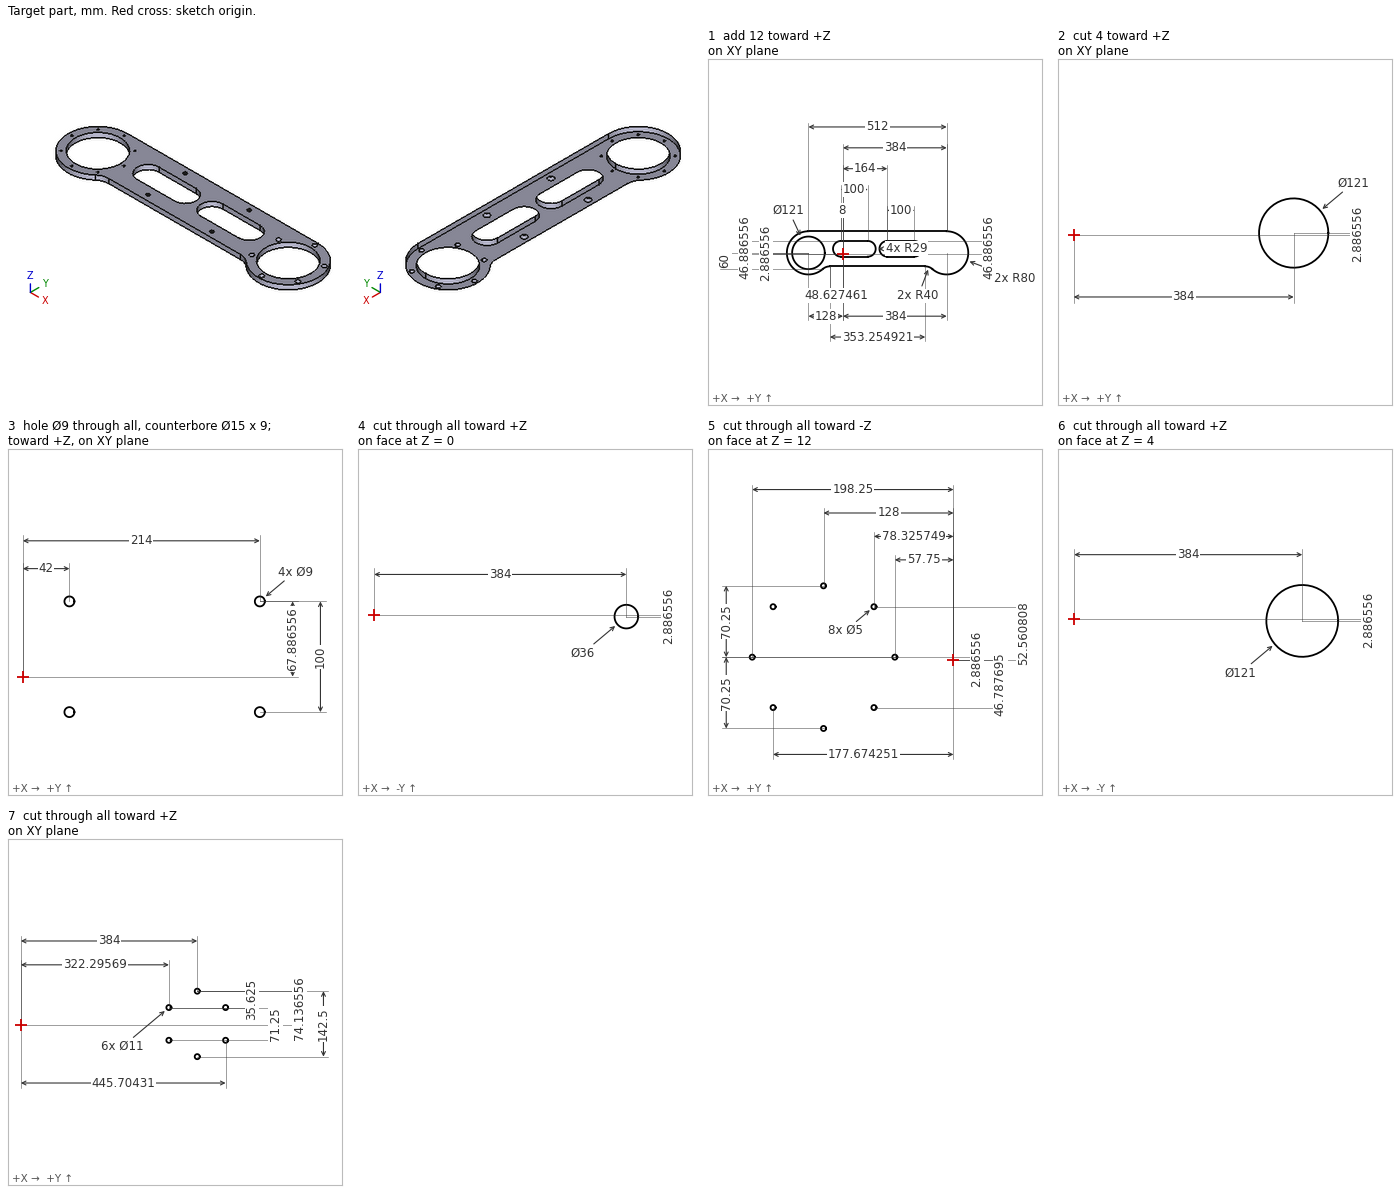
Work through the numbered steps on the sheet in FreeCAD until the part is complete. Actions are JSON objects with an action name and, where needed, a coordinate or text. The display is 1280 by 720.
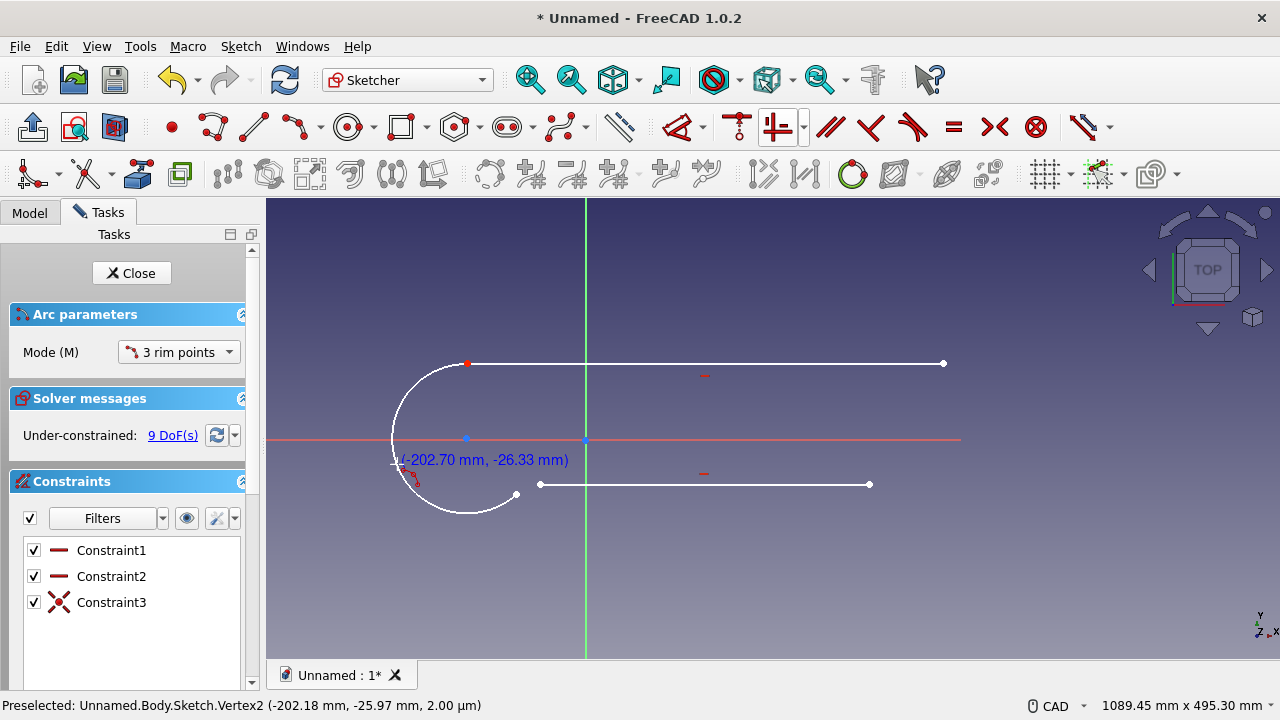
{"action": "left_click", "coordinate": [516, 495]}
{"action": "left_click", "coordinate": [540, 485]}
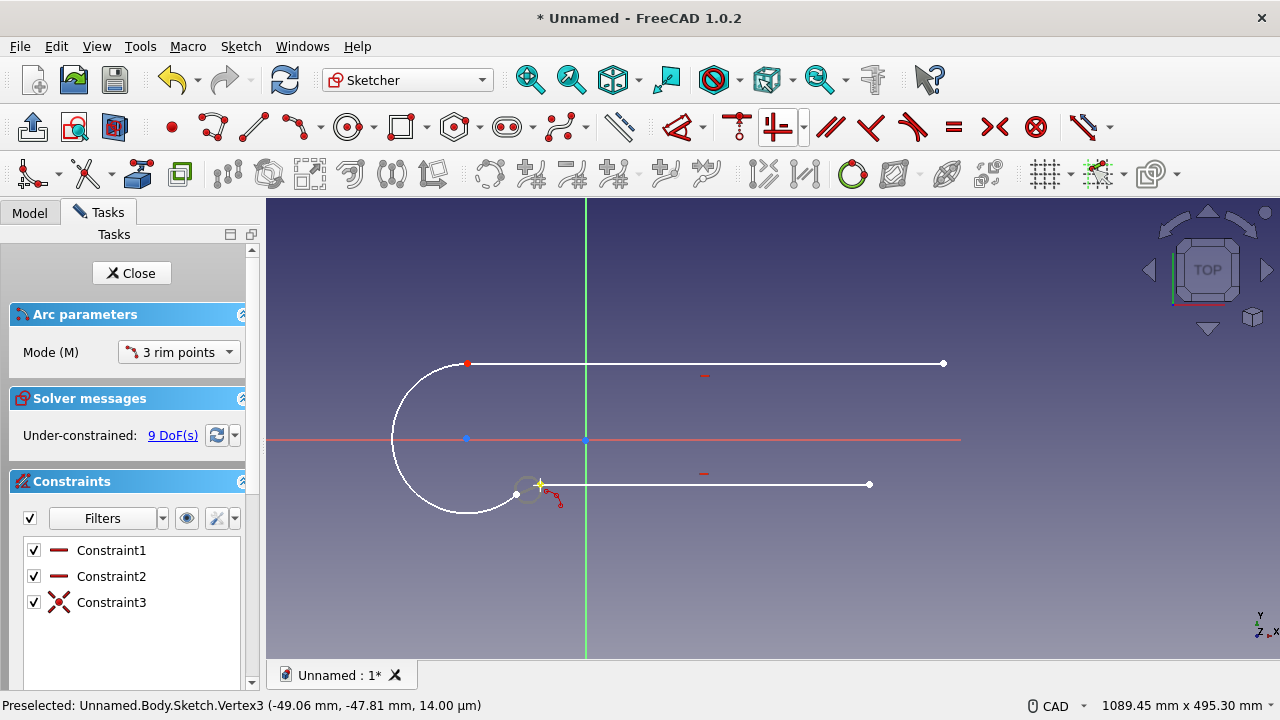
{"action": "scroll", "coordinate": [527, 487], "scroll_direction": "up", "scroll_amount": 10}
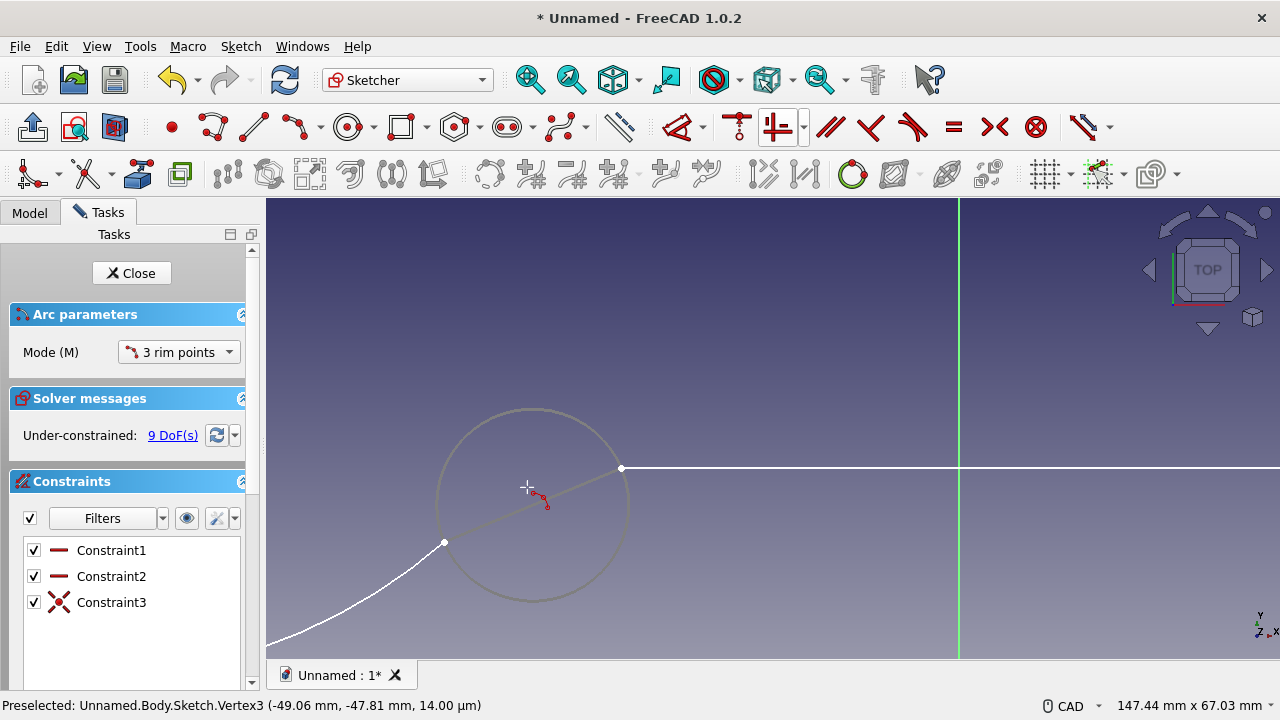
{"action": "left_click", "coordinate": [527, 481]}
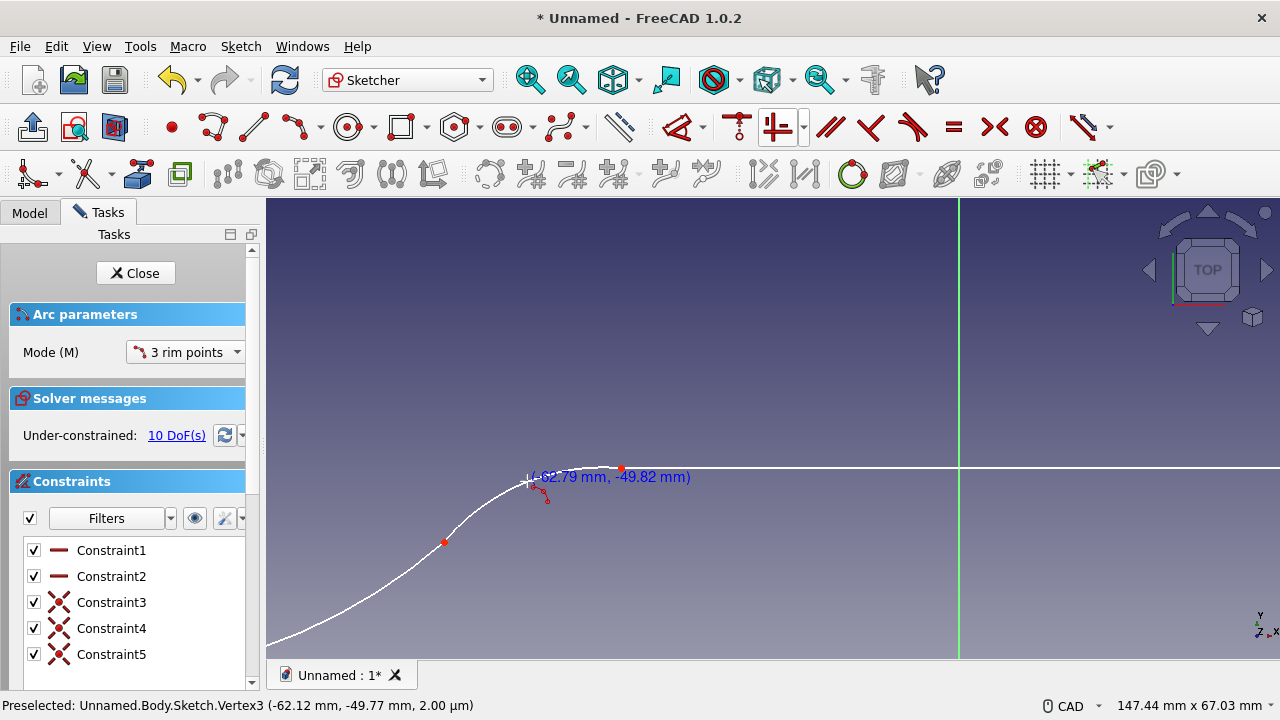
{"action": "scroll", "coordinate": [527, 487], "scroll_direction": "down", "scroll_amount": 10}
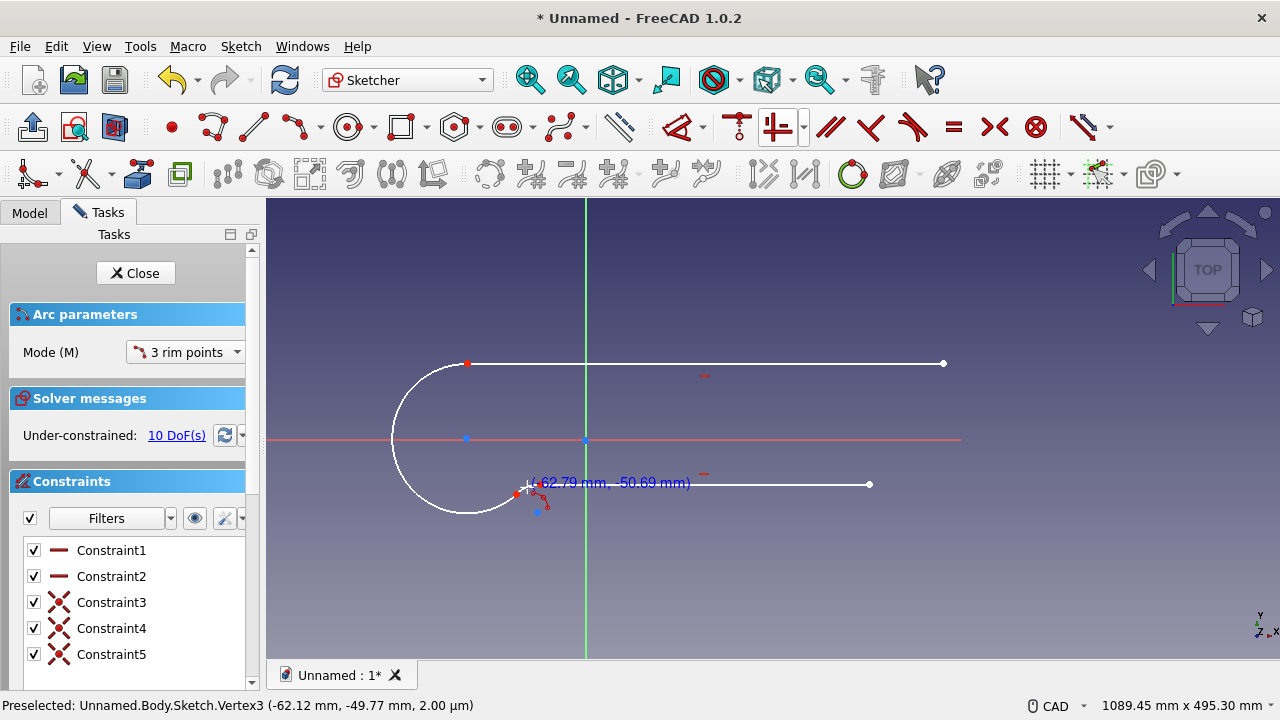
{"action": "left_click", "coordinate": [869, 485]}
{"action": "left_click", "coordinate": [894, 494]}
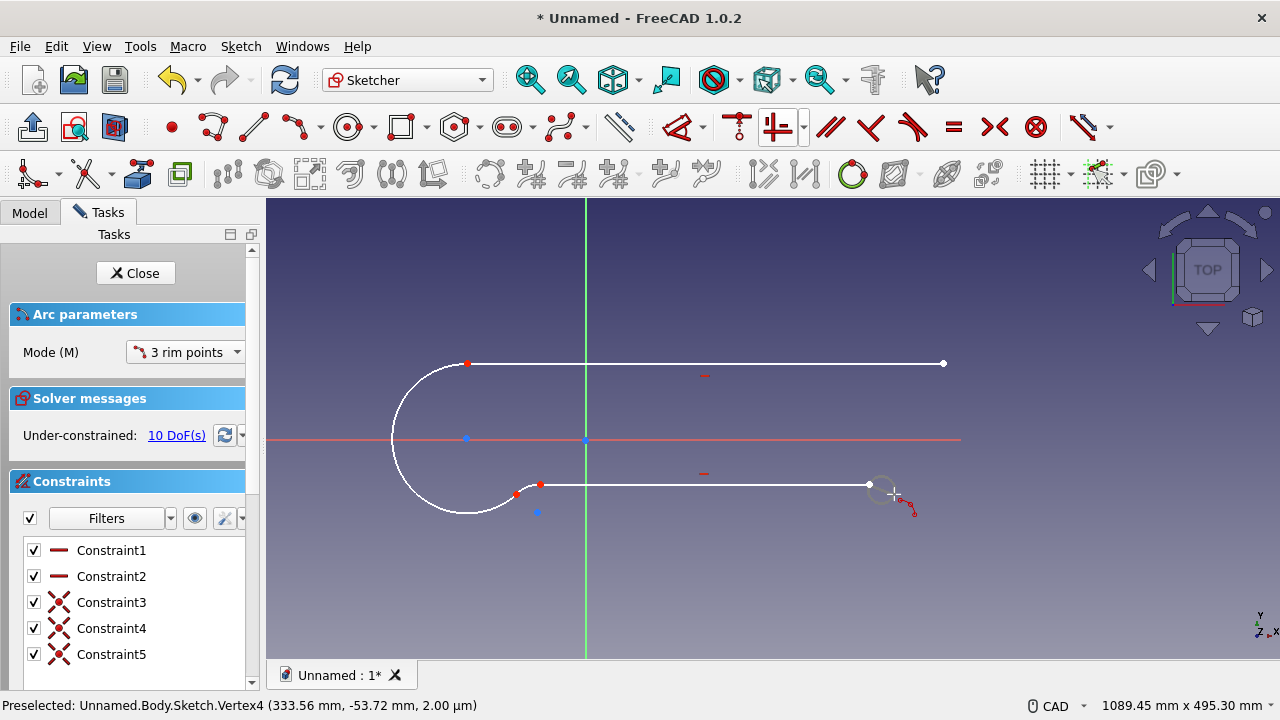
{"action": "scroll", "coordinate": [882, 487], "scroll_direction": "up", "scroll_amount": 10}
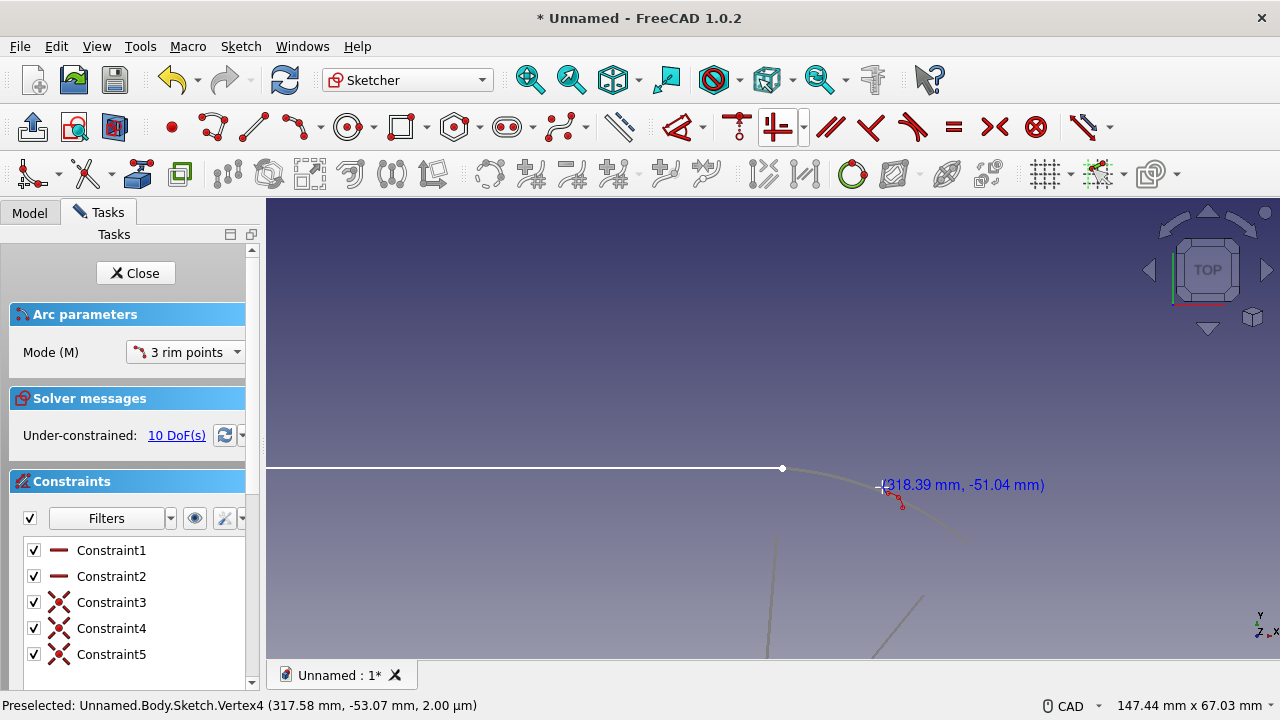
{"action": "left_click", "coordinate": [881, 481]}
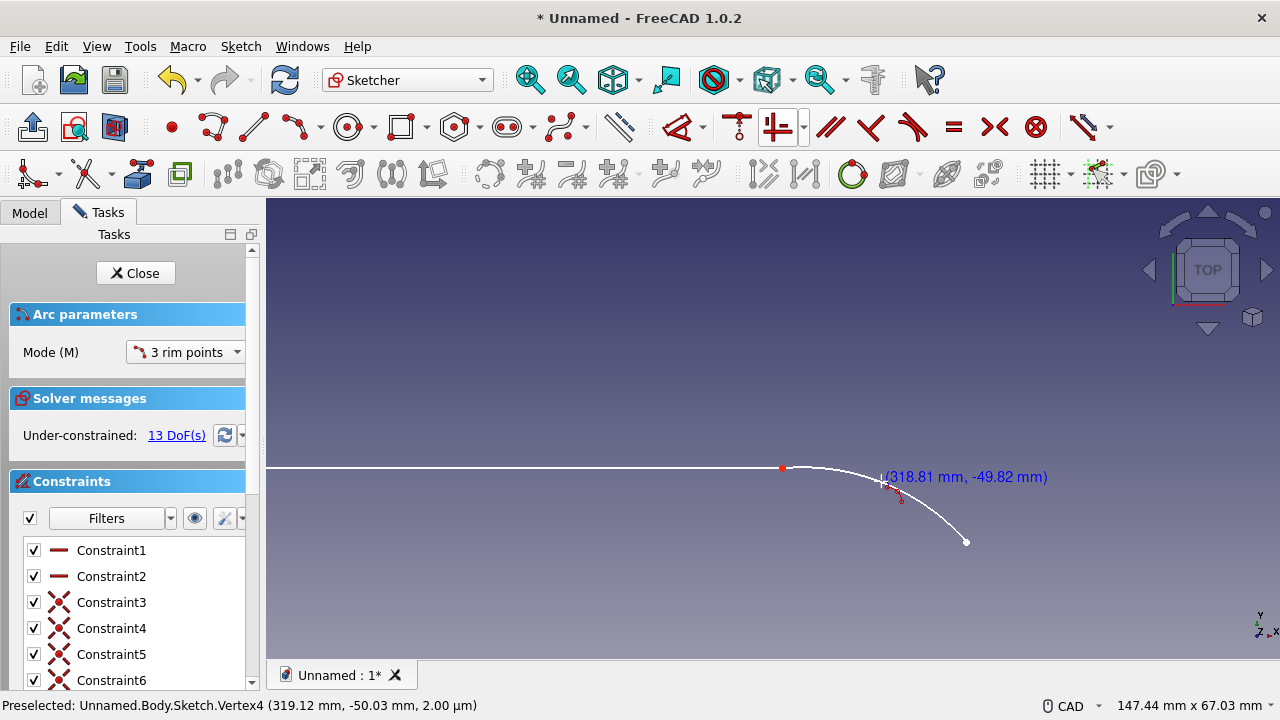
{"action": "scroll", "coordinate": [882, 487], "scroll_direction": "down", "scroll_amount": 10}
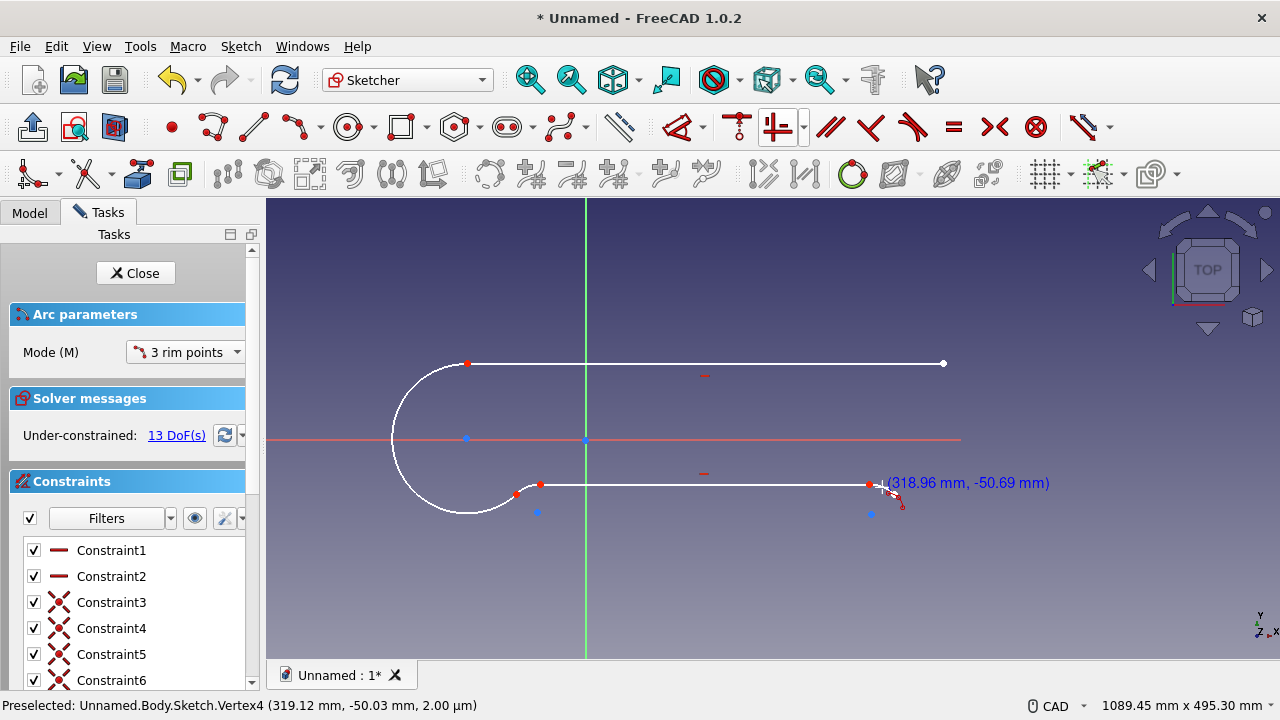
{"action": "left_click", "coordinate": [894, 495]}
{"action": "left_click", "coordinate": [943, 364]}
{"action": "left_click", "coordinate": [1013, 464]}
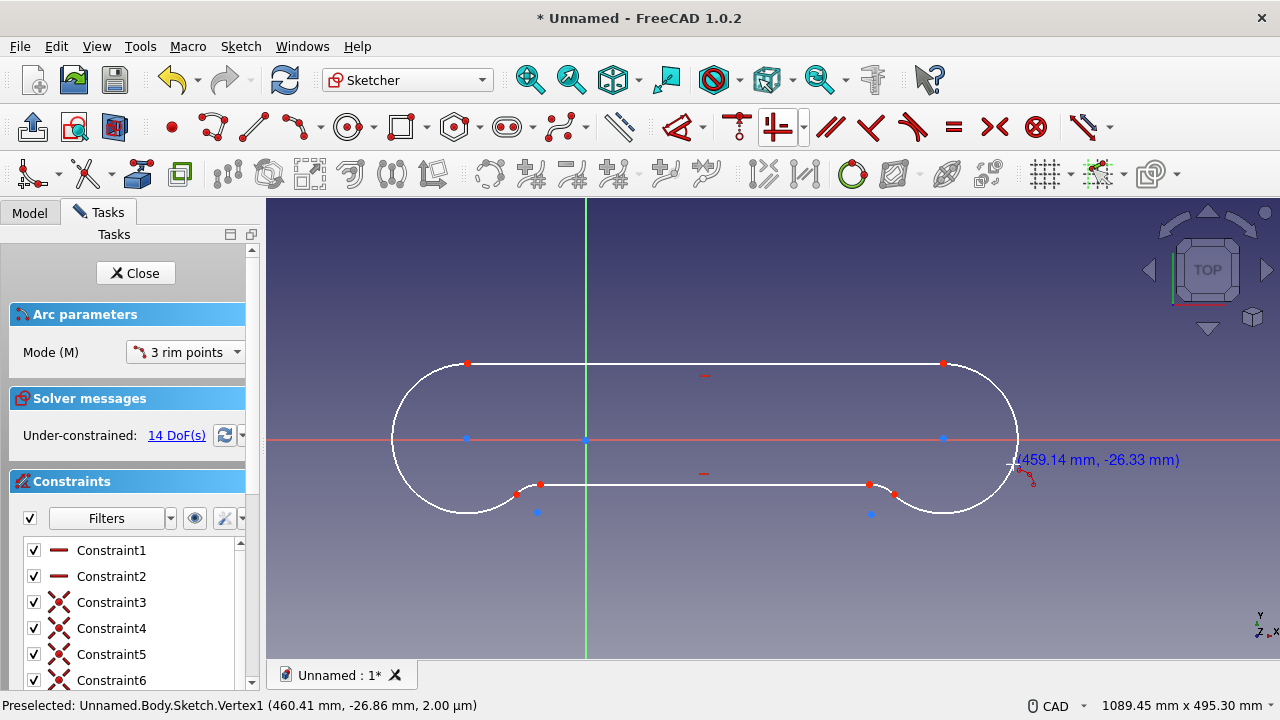
{"action": "left_click", "coordinate": [506, 128]}